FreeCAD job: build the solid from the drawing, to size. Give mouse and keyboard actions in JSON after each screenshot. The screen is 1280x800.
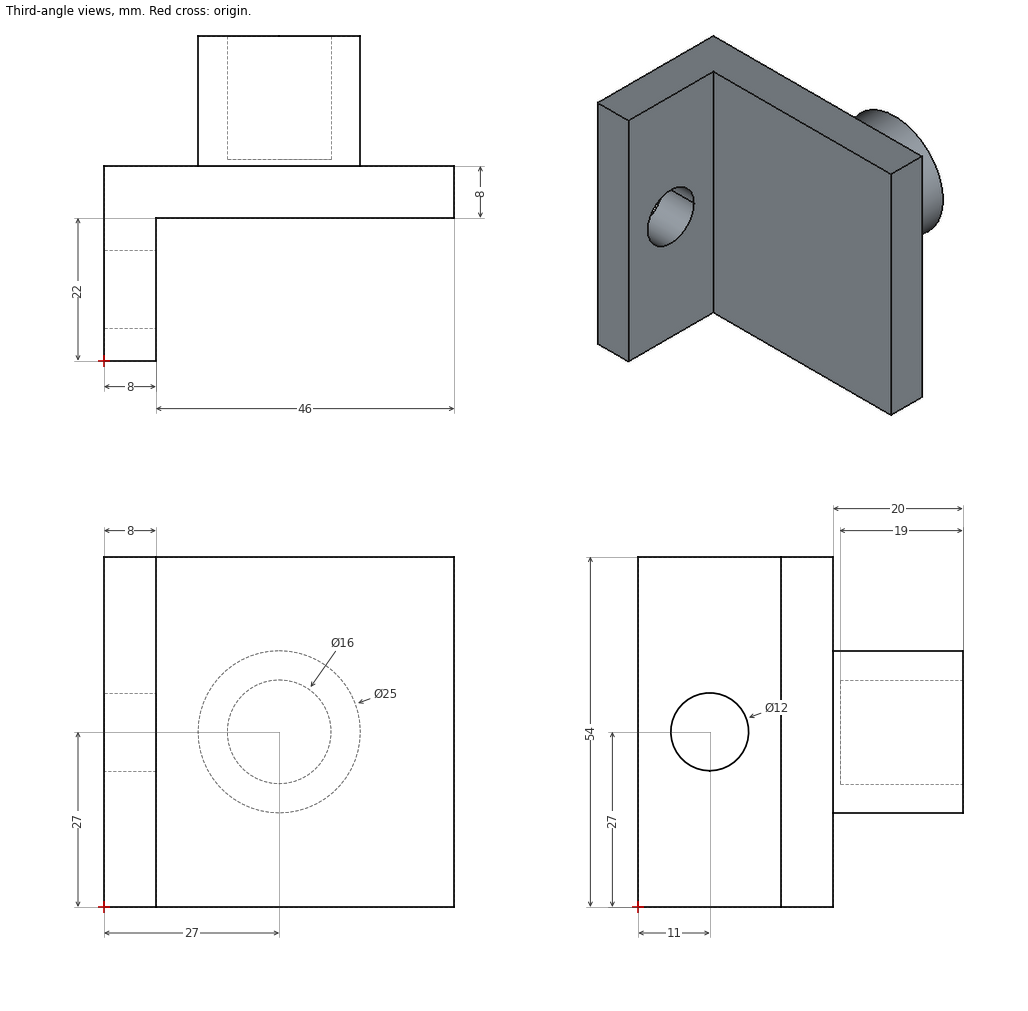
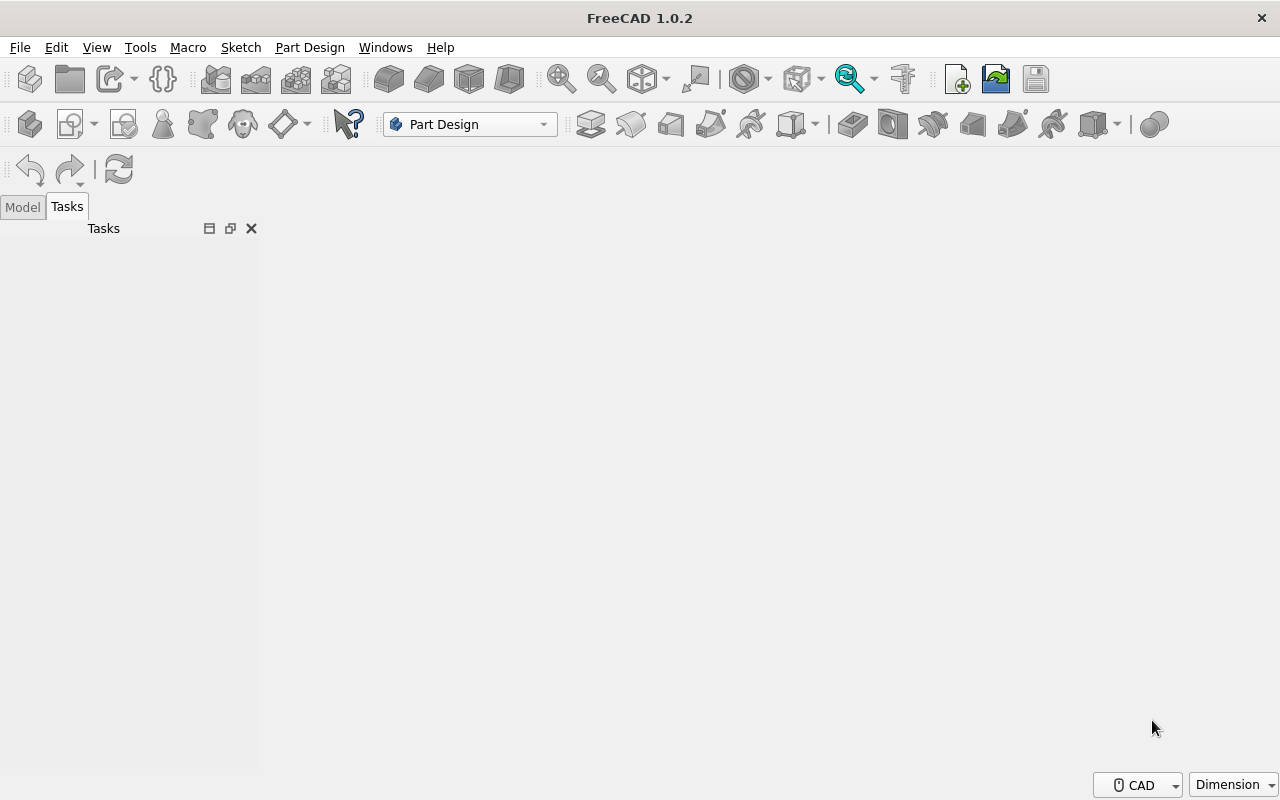
{"action": "left_click", "coordinate": [956, 80]}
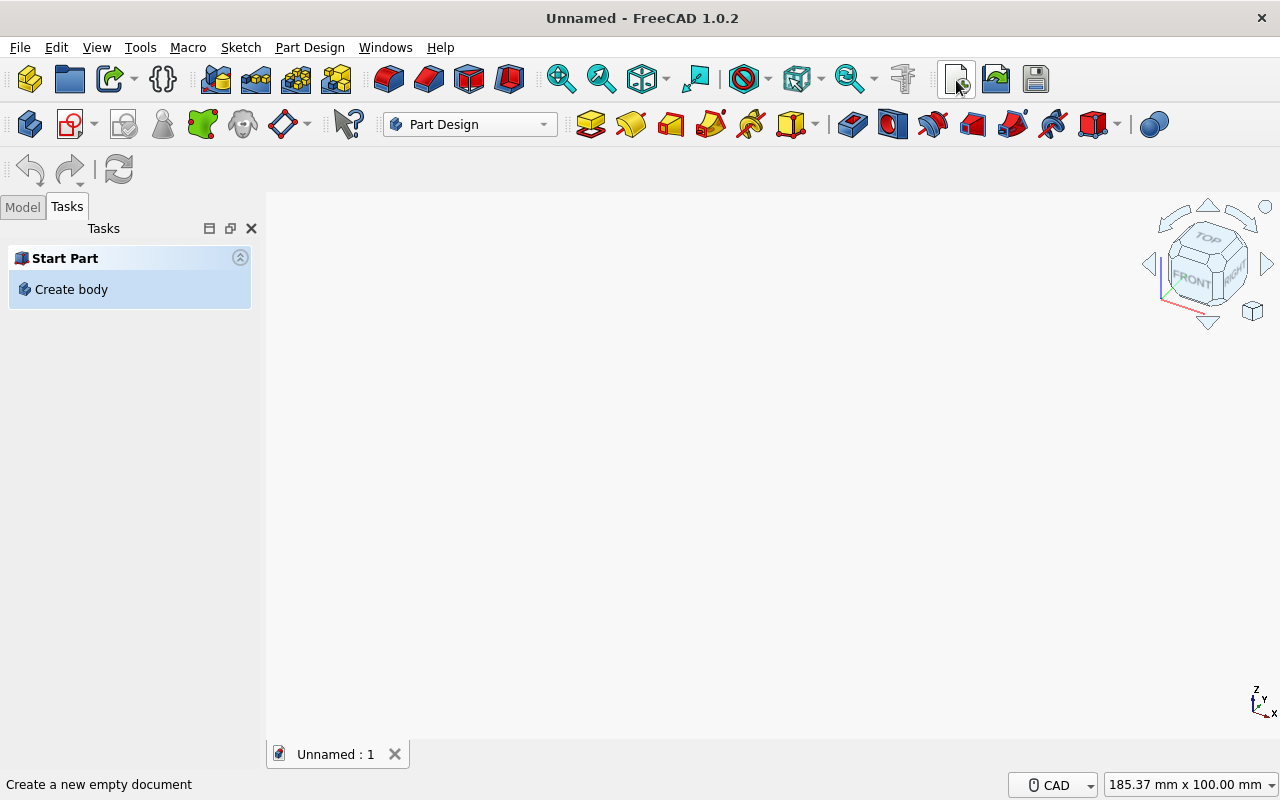
{"action": "left_click", "coordinate": [70, 124]}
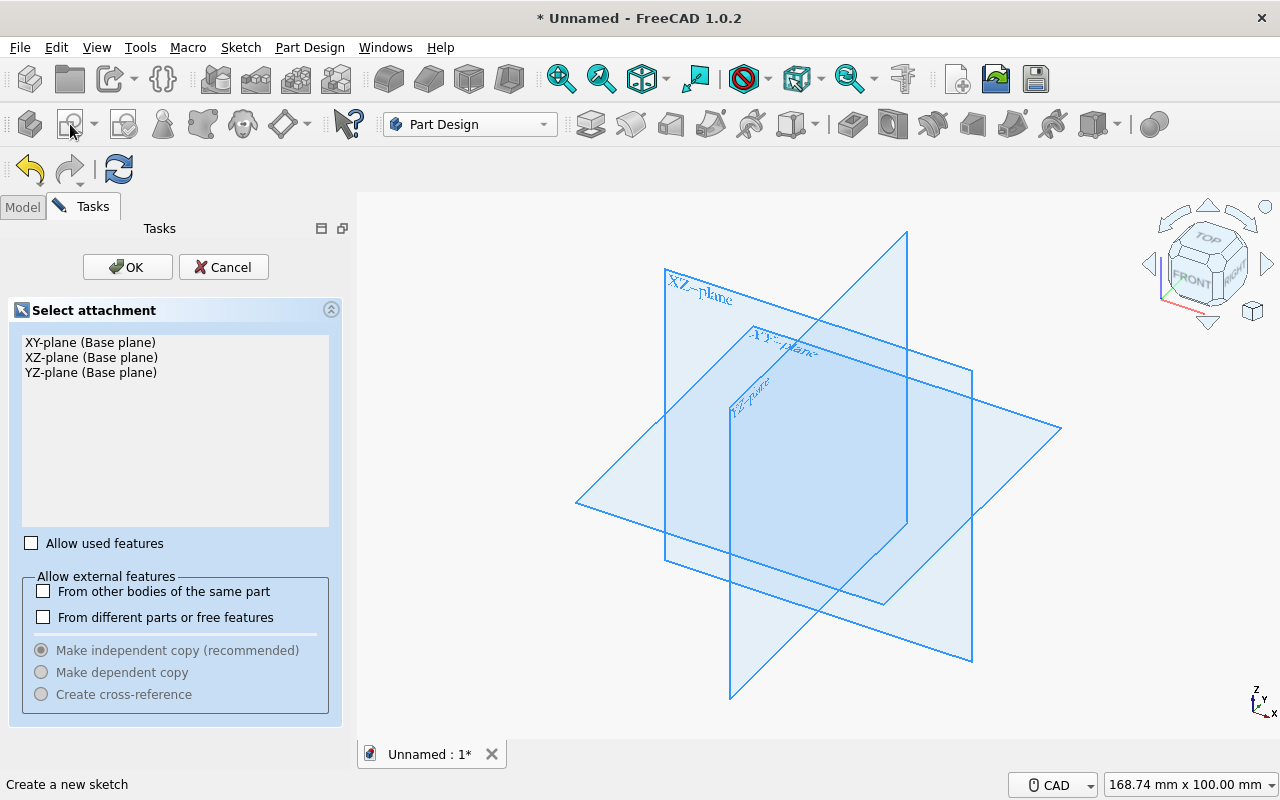
{"action": "left_click", "coordinate": [82, 342]}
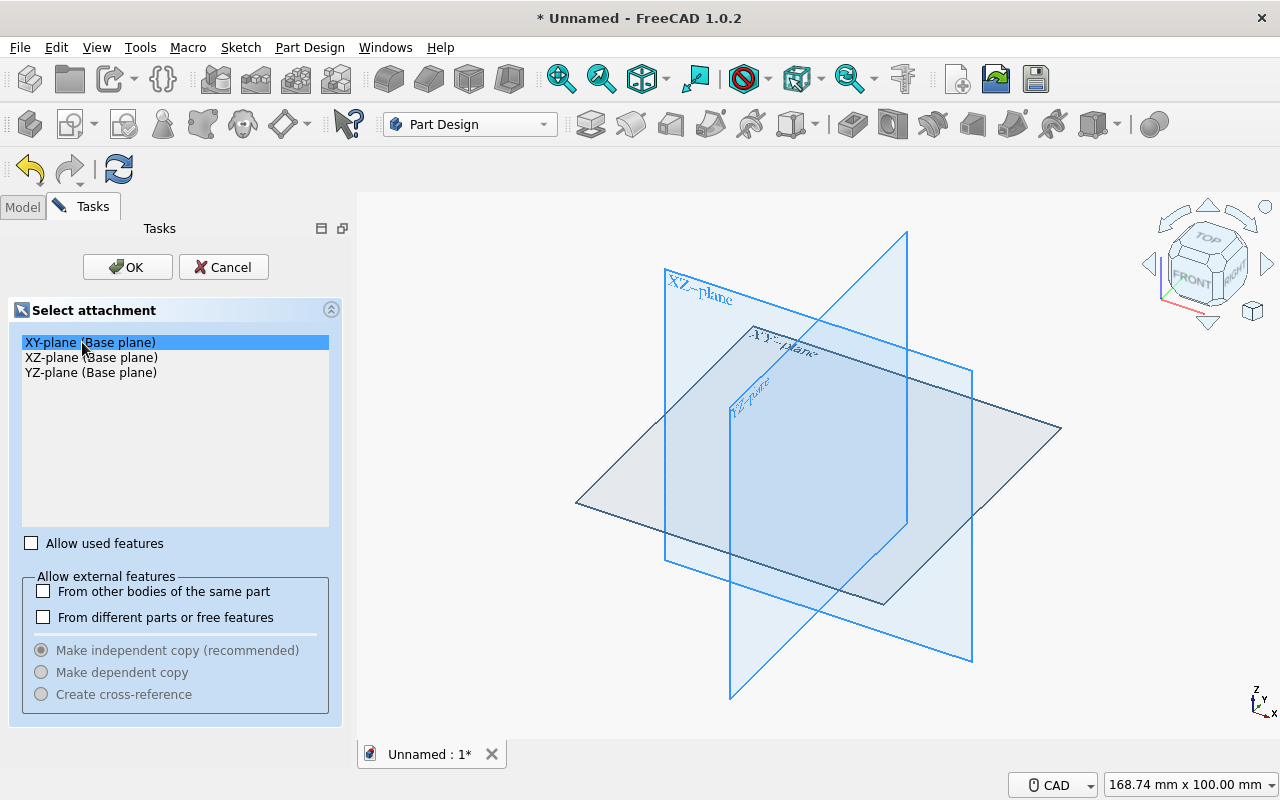
{"action": "left_click", "coordinate": [128, 267]}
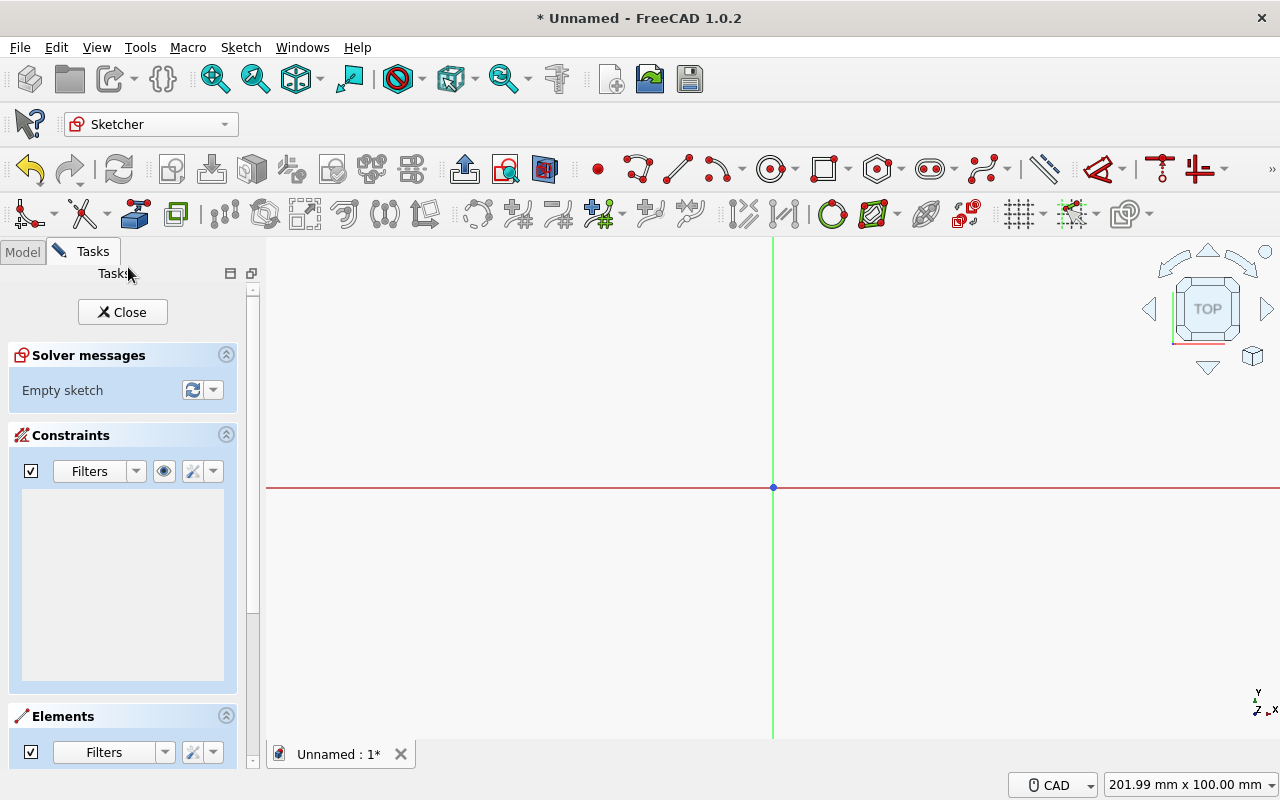
{"action": "scroll", "coordinate": [1075, 351], "scroll_direction": "up", "scroll_amount": 4}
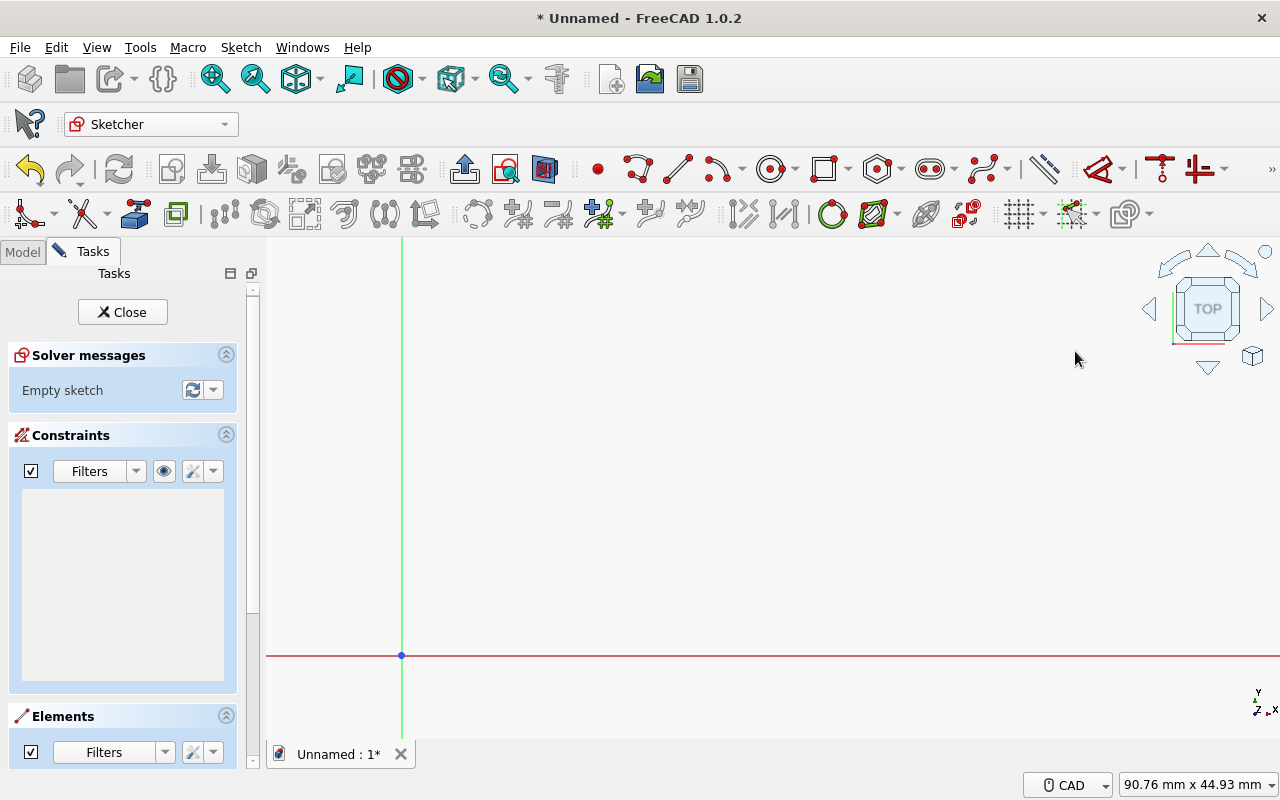
{"action": "key", "text": "g m"}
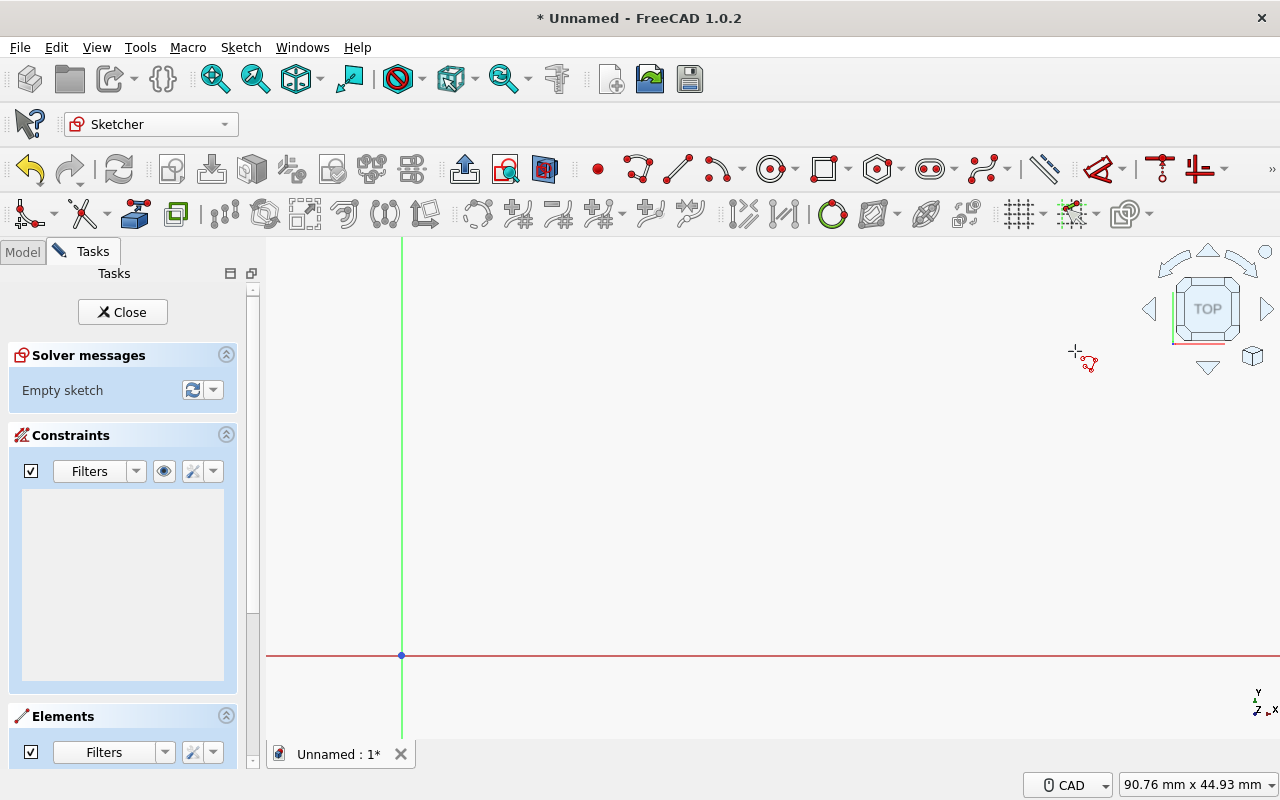
{"action": "left_click", "coordinate": [402, 656]}
{"action": "left_click", "coordinate": [491, 647]}
{"action": "left_click", "coordinate": [491, 410]}
{"action": "left_click", "coordinate": [1005, 410]}
{"action": "left_click", "coordinate": [1005, 320]}
{"action": "left_click", "coordinate": [411, 320]}
{"action": "left_click", "coordinate": [402, 656]}
{"action": "key", "text": "Escape"}
{"action": "key", "text": "Escape"}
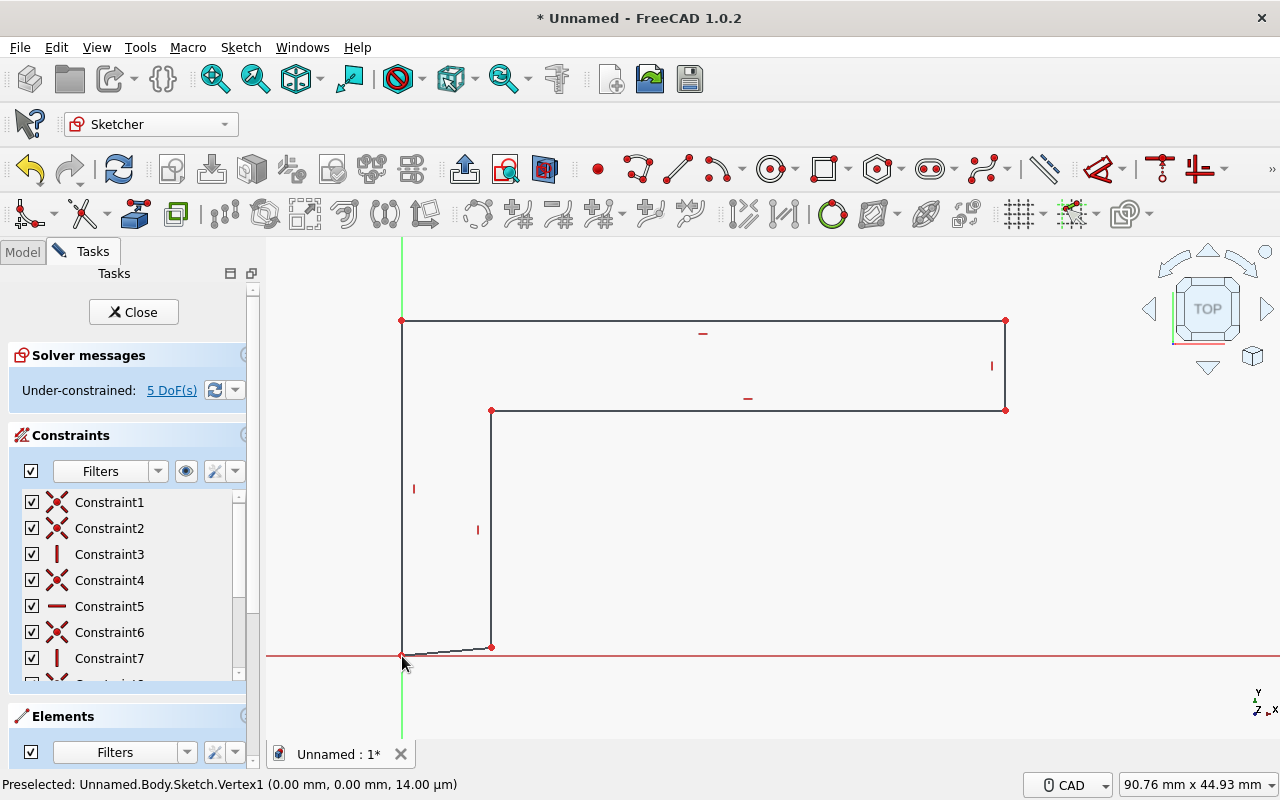
{"action": "left_click", "coordinate": [429, 653]}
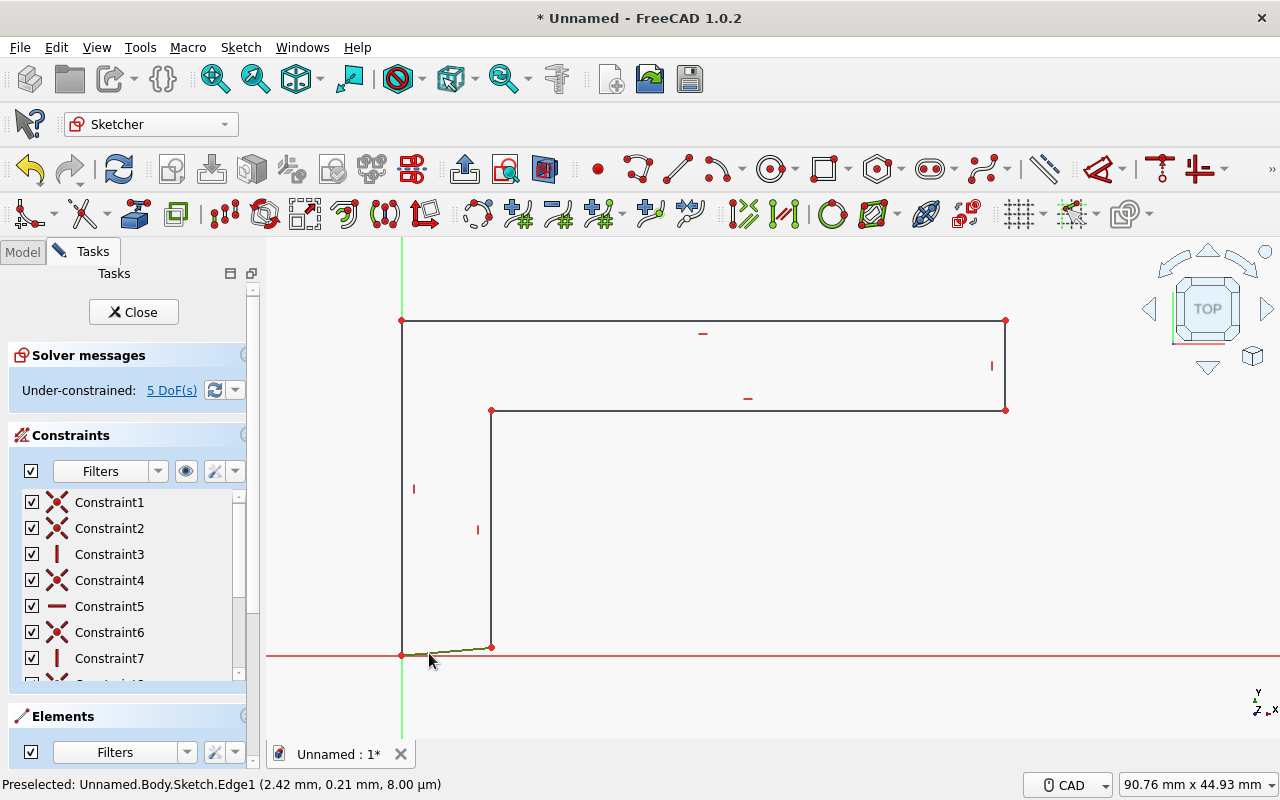
{"action": "key", "text": "h"}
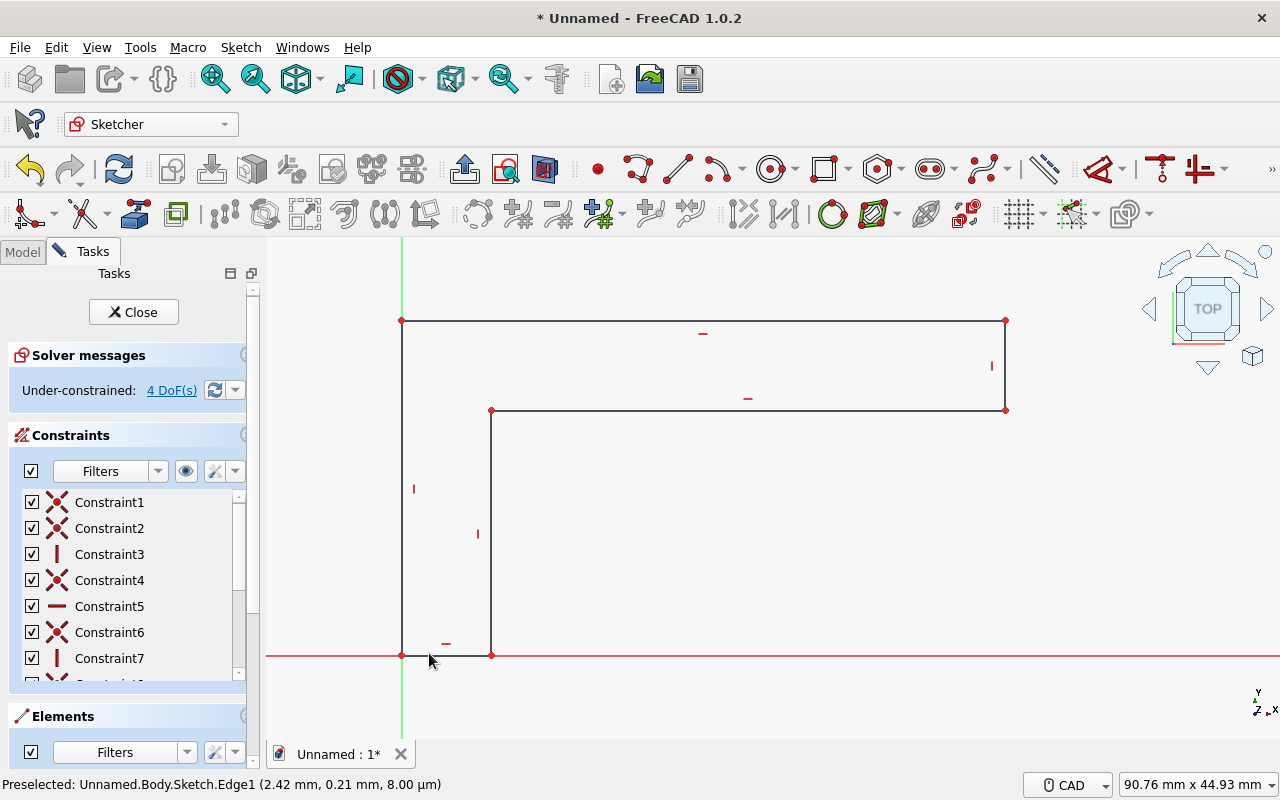
{"action": "left_click", "coordinate": [429, 656]}